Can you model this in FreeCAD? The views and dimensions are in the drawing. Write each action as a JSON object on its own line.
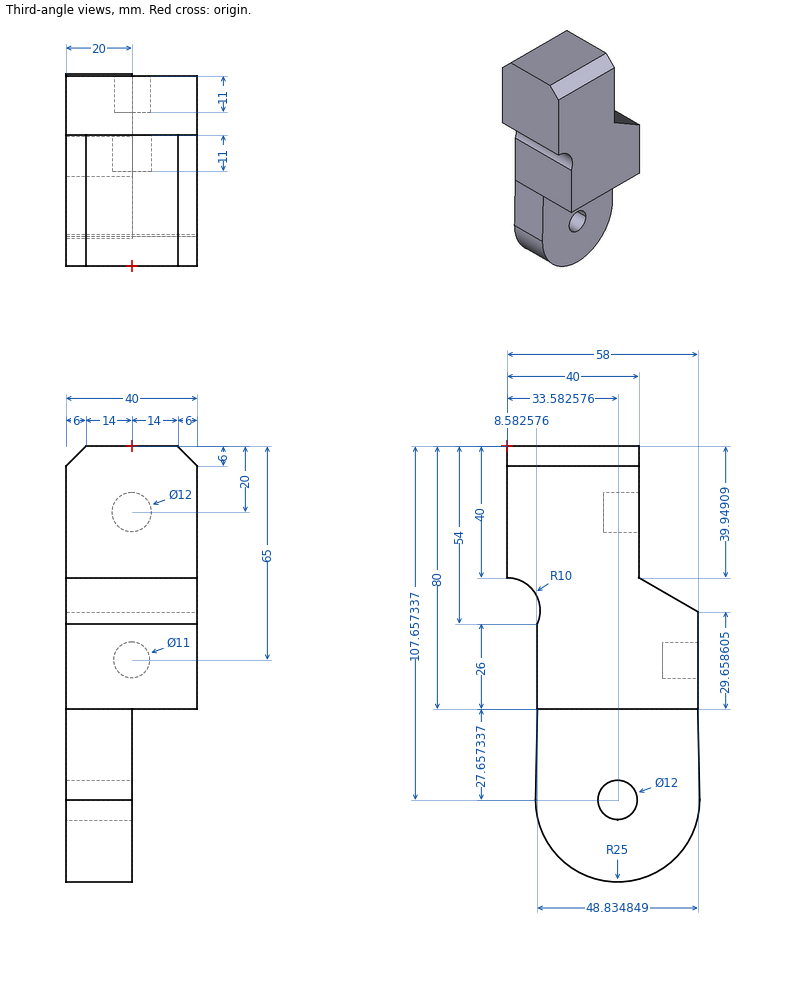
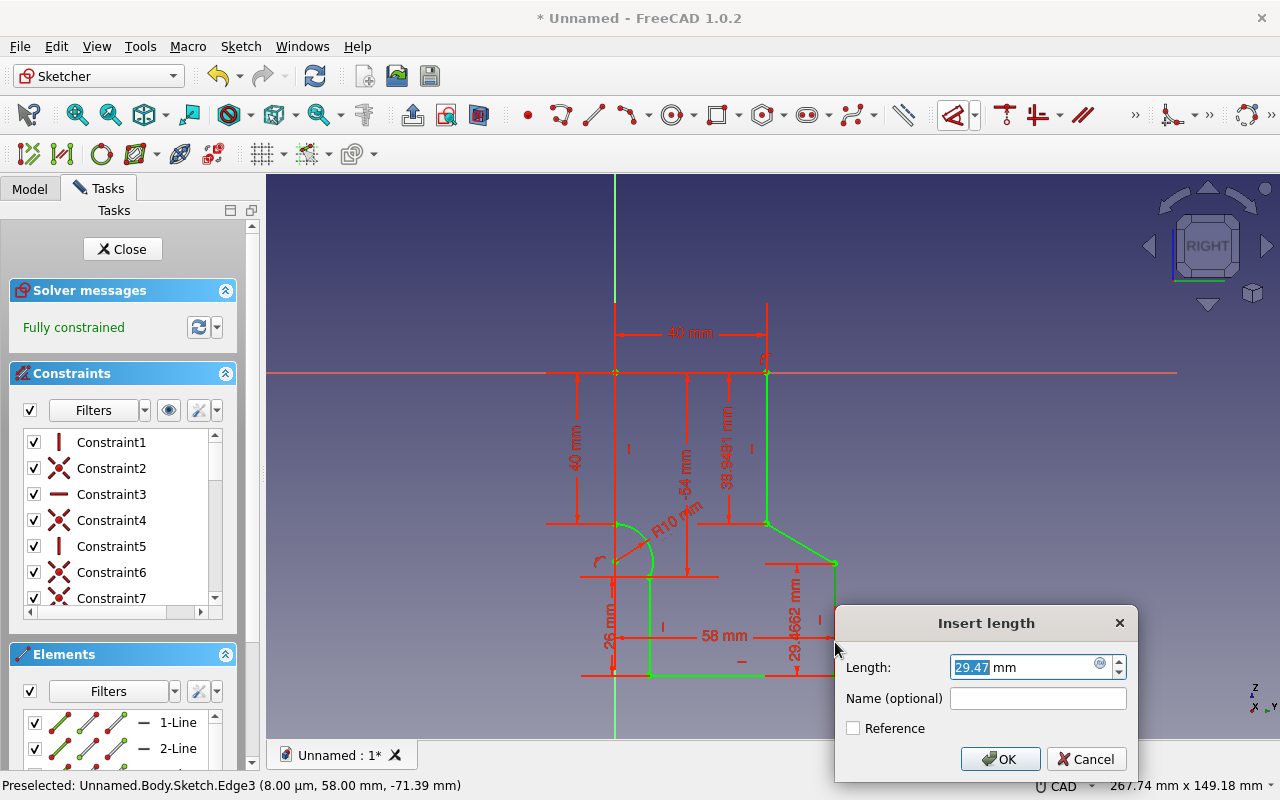
{"action": "type", "text": "29.658605"}
{"action": "key", "text": "Return"}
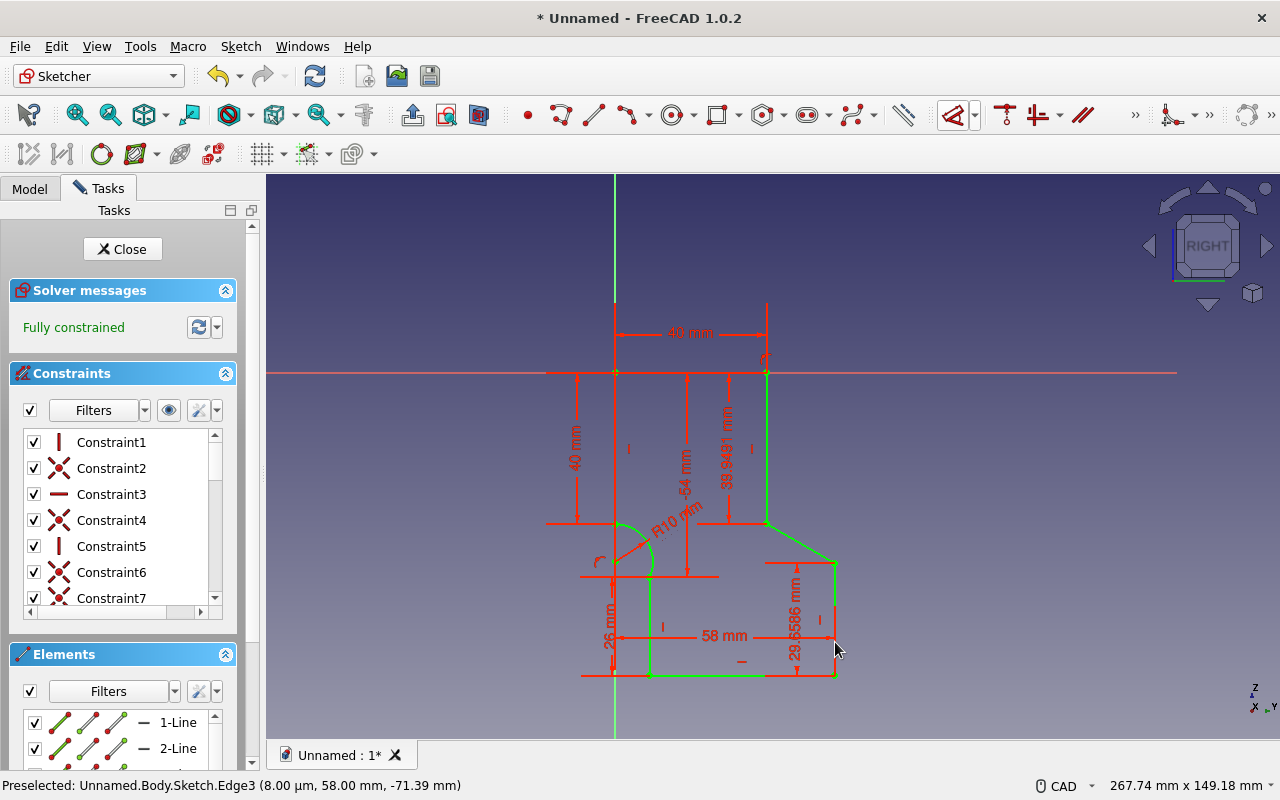
{"action": "left_click", "coordinate": [123, 249]}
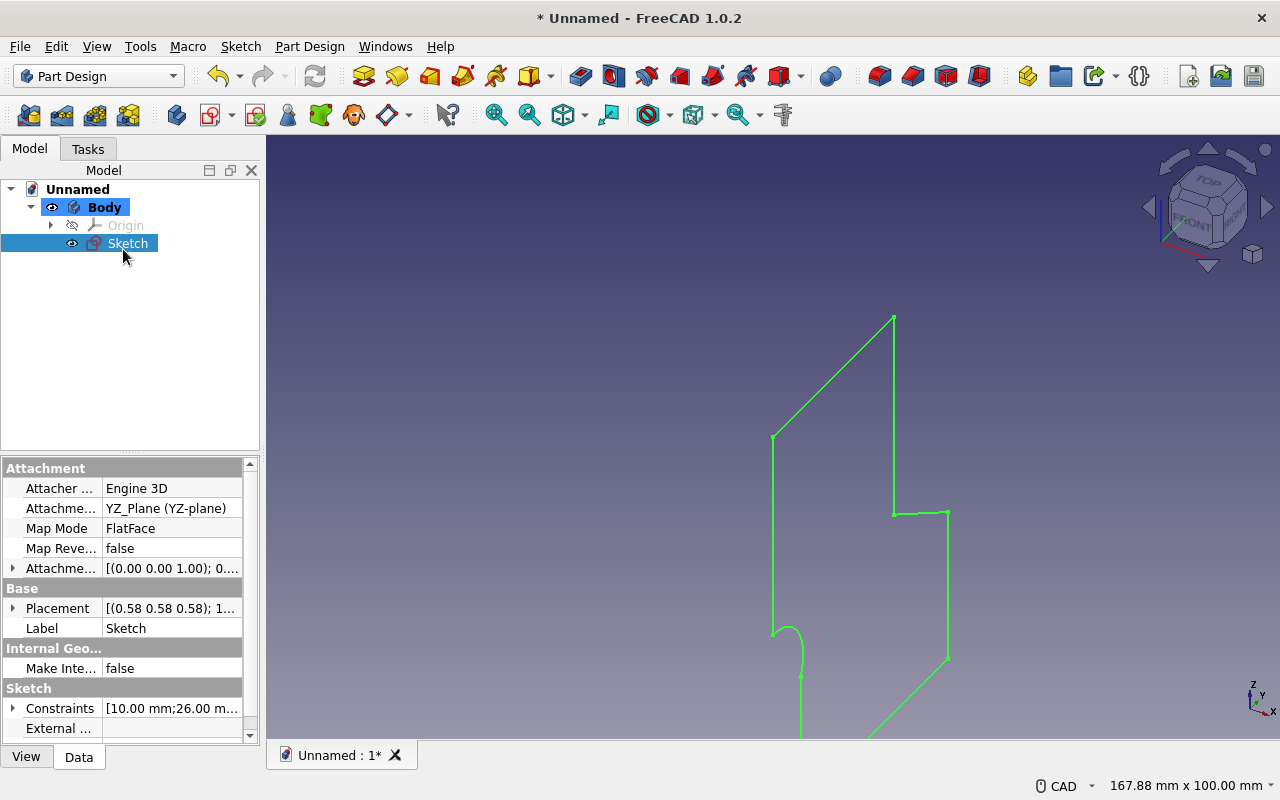
{"action": "left_click", "coordinate": [364, 76]}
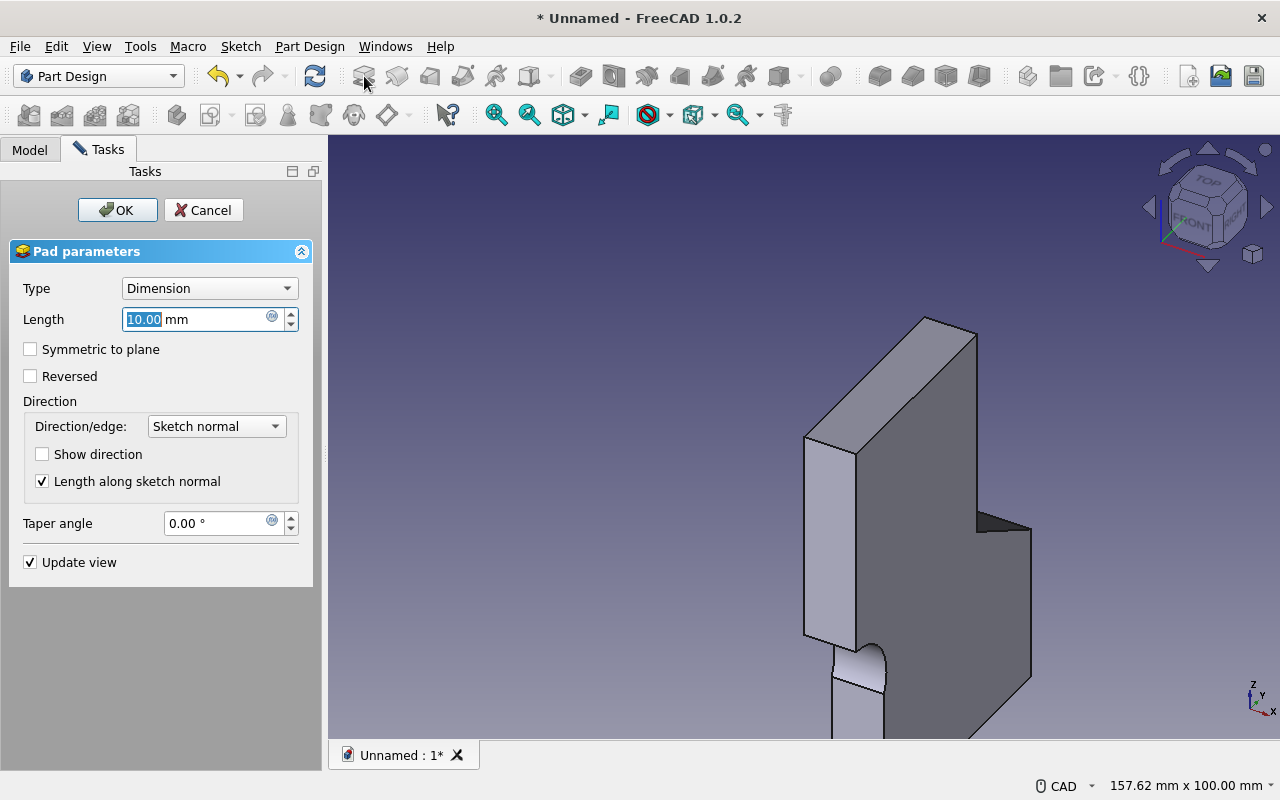
{"action": "type", "text": "40"}
{"action": "key", "text": "Tab"}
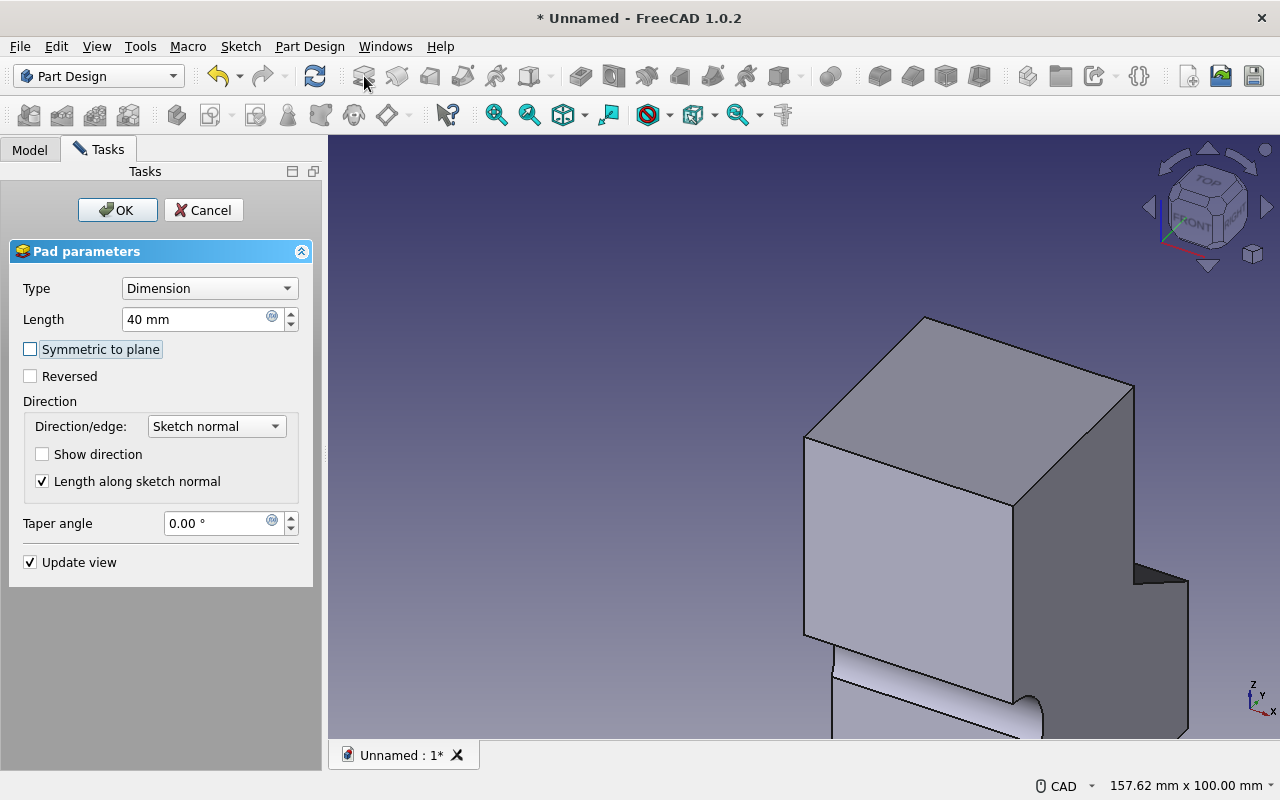
{"action": "left_click", "coordinate": [31, 349]}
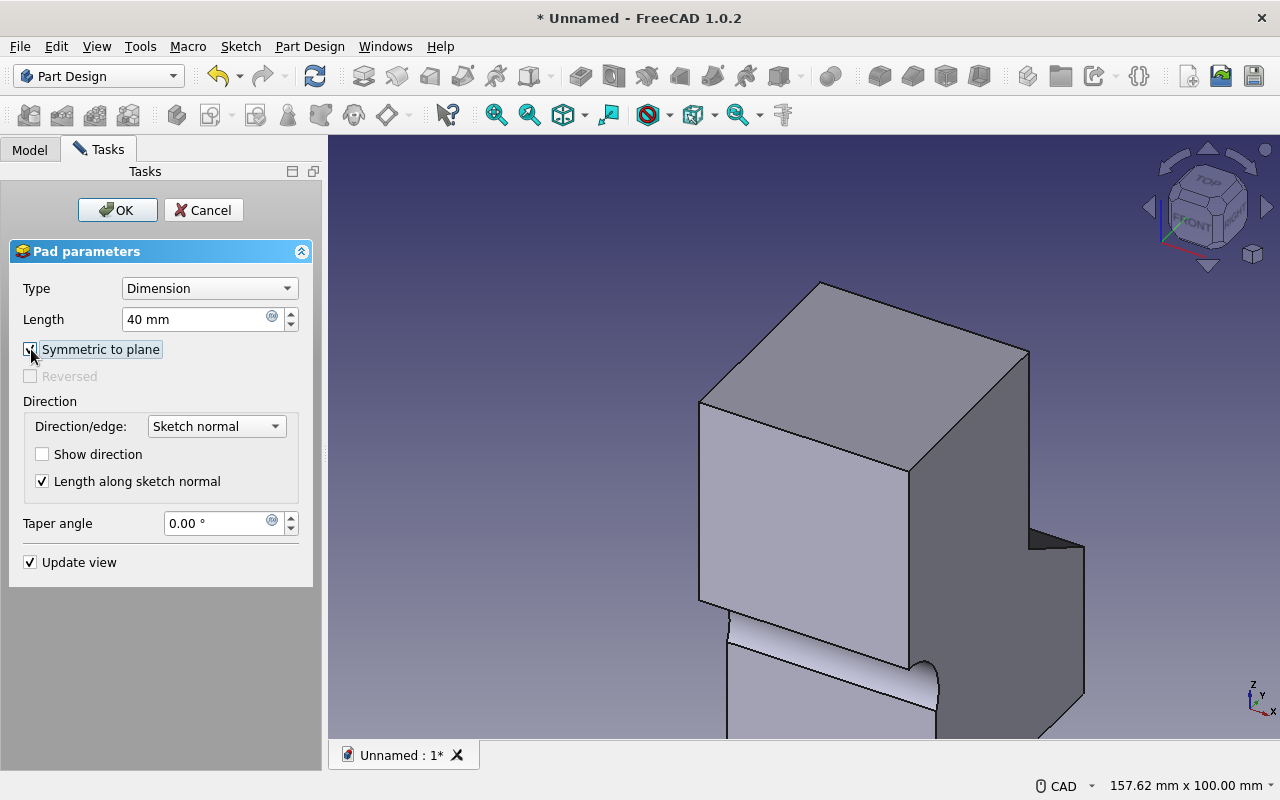
{"action": "left_click", "coordinate": [118, 210]}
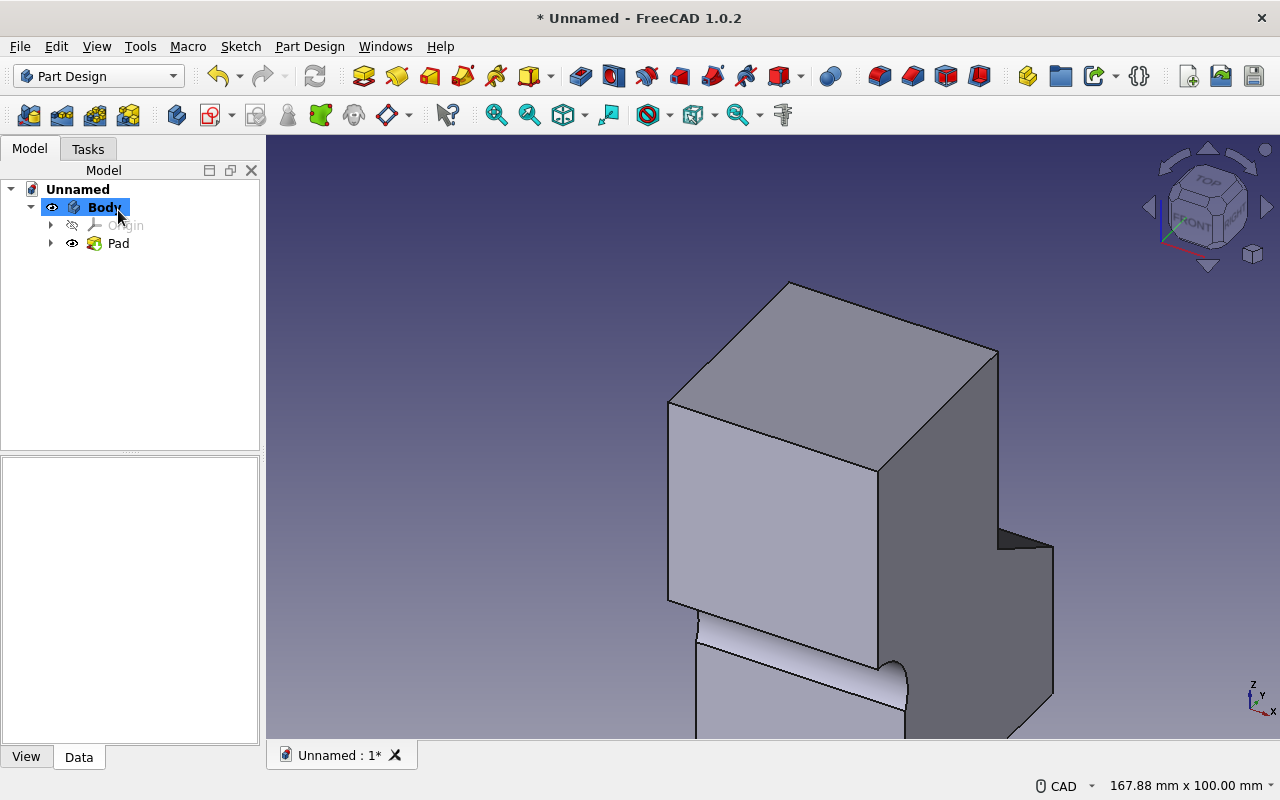
{"action": "key", "text": "v f"}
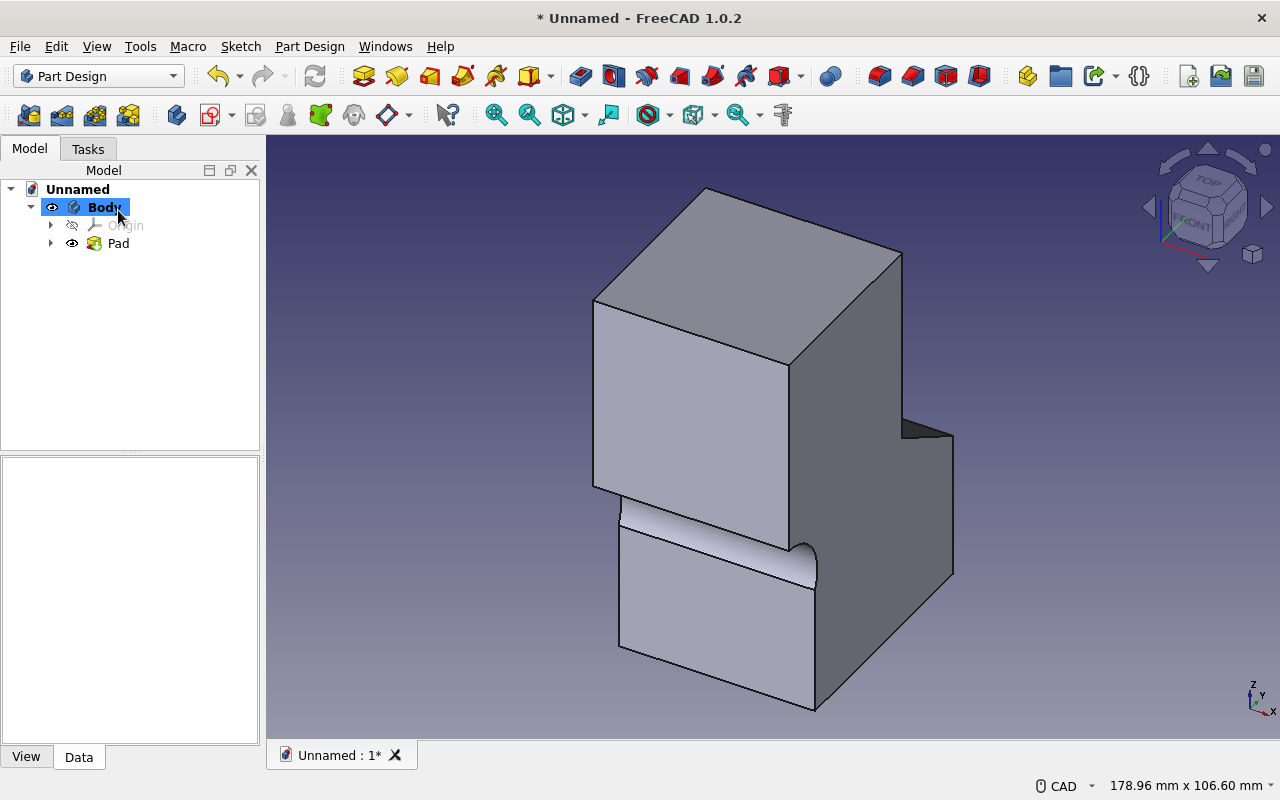
{"action": "left_click", "coordinate": [691, 425]}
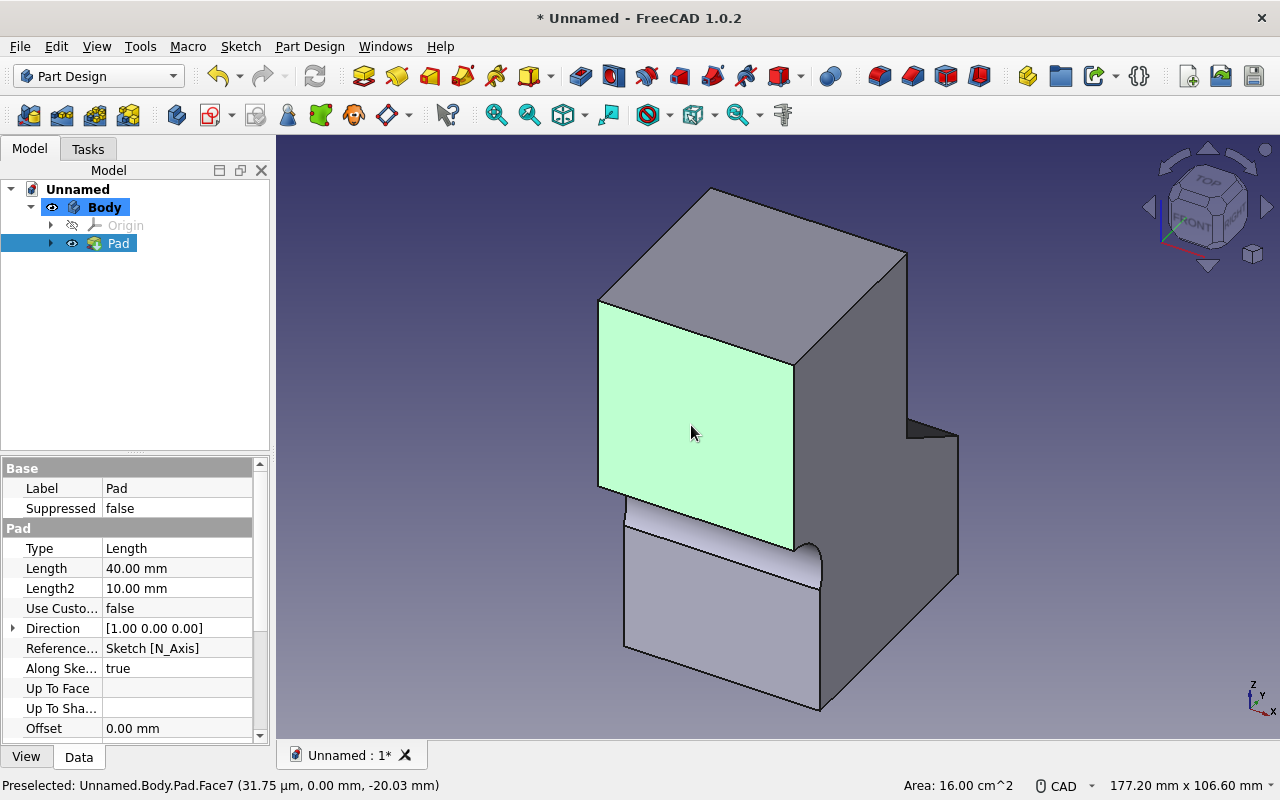
{"action": "left_click", "coordinate": [210, 116]}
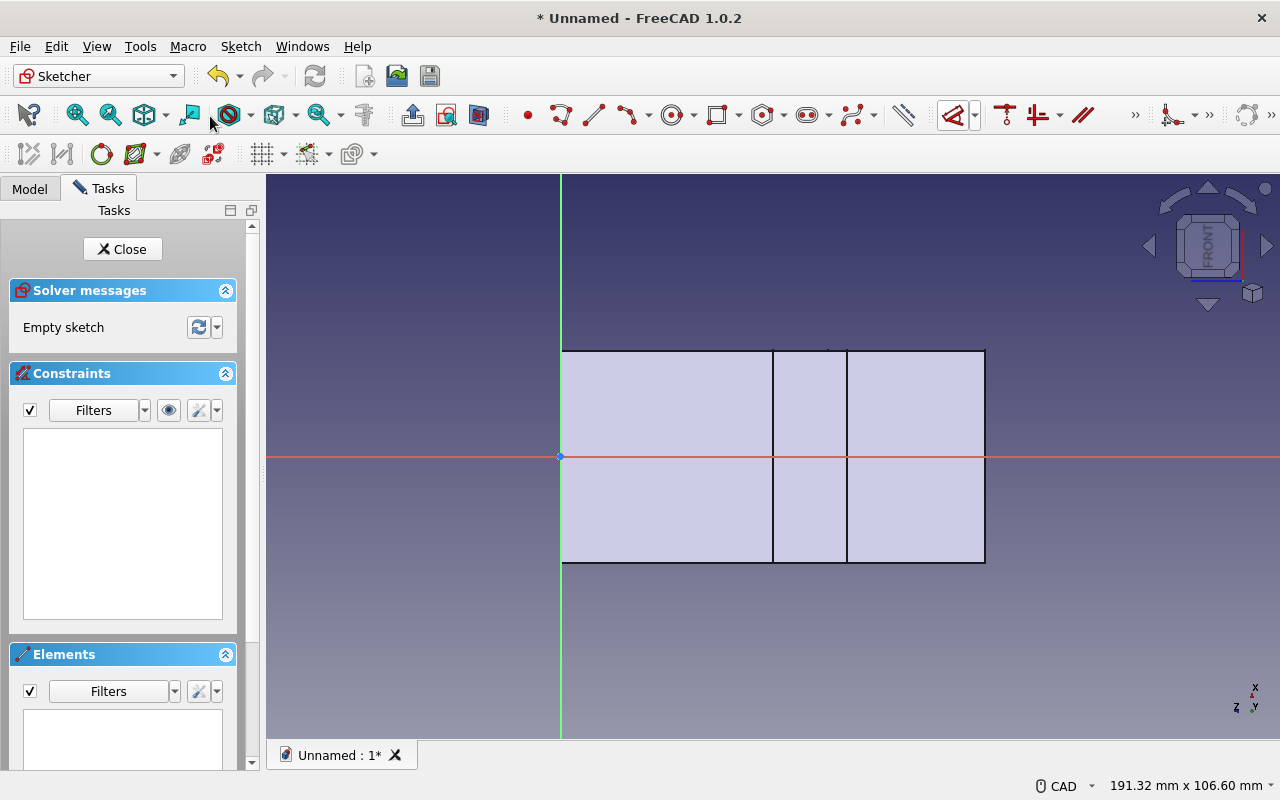
{"action": "scroll", "coordinate": [564, 357], "scroll_direction": "up", "scroll_amount": 12}